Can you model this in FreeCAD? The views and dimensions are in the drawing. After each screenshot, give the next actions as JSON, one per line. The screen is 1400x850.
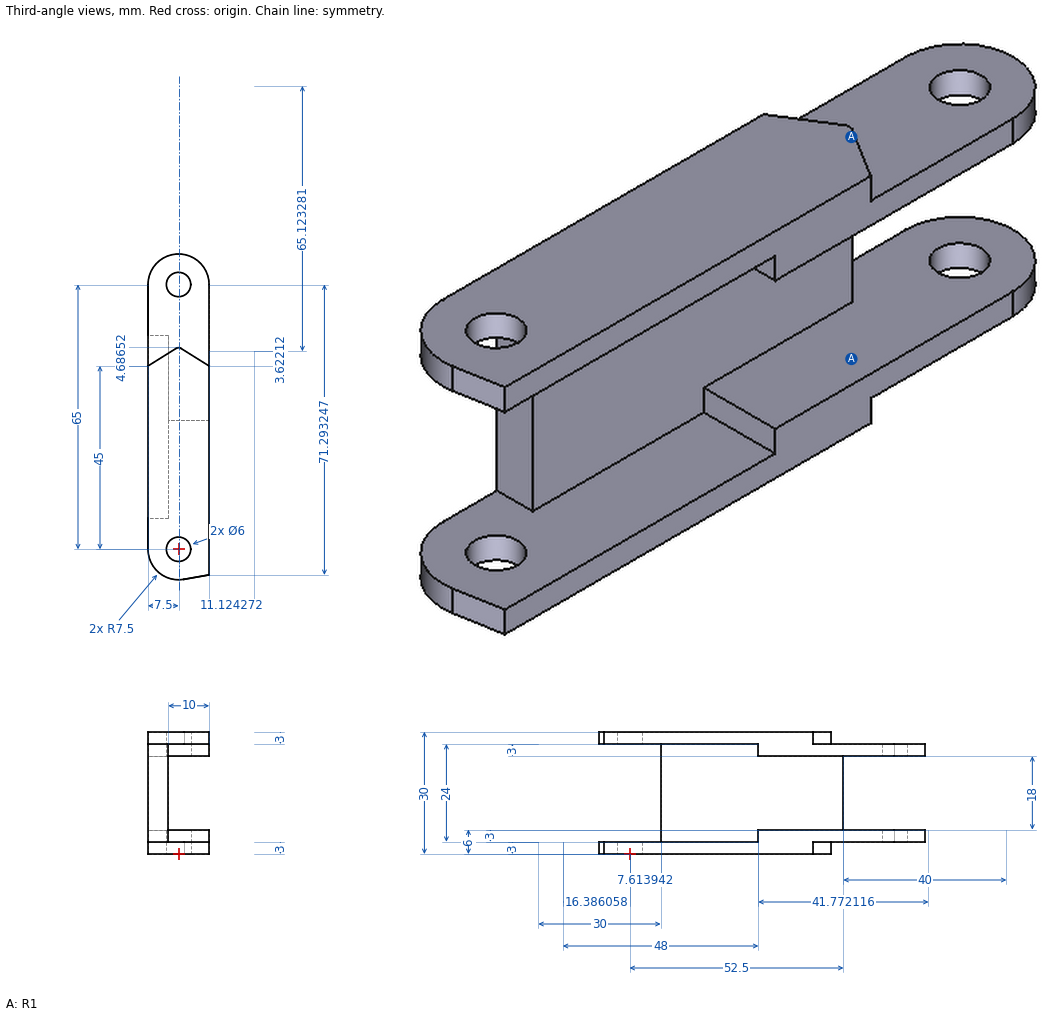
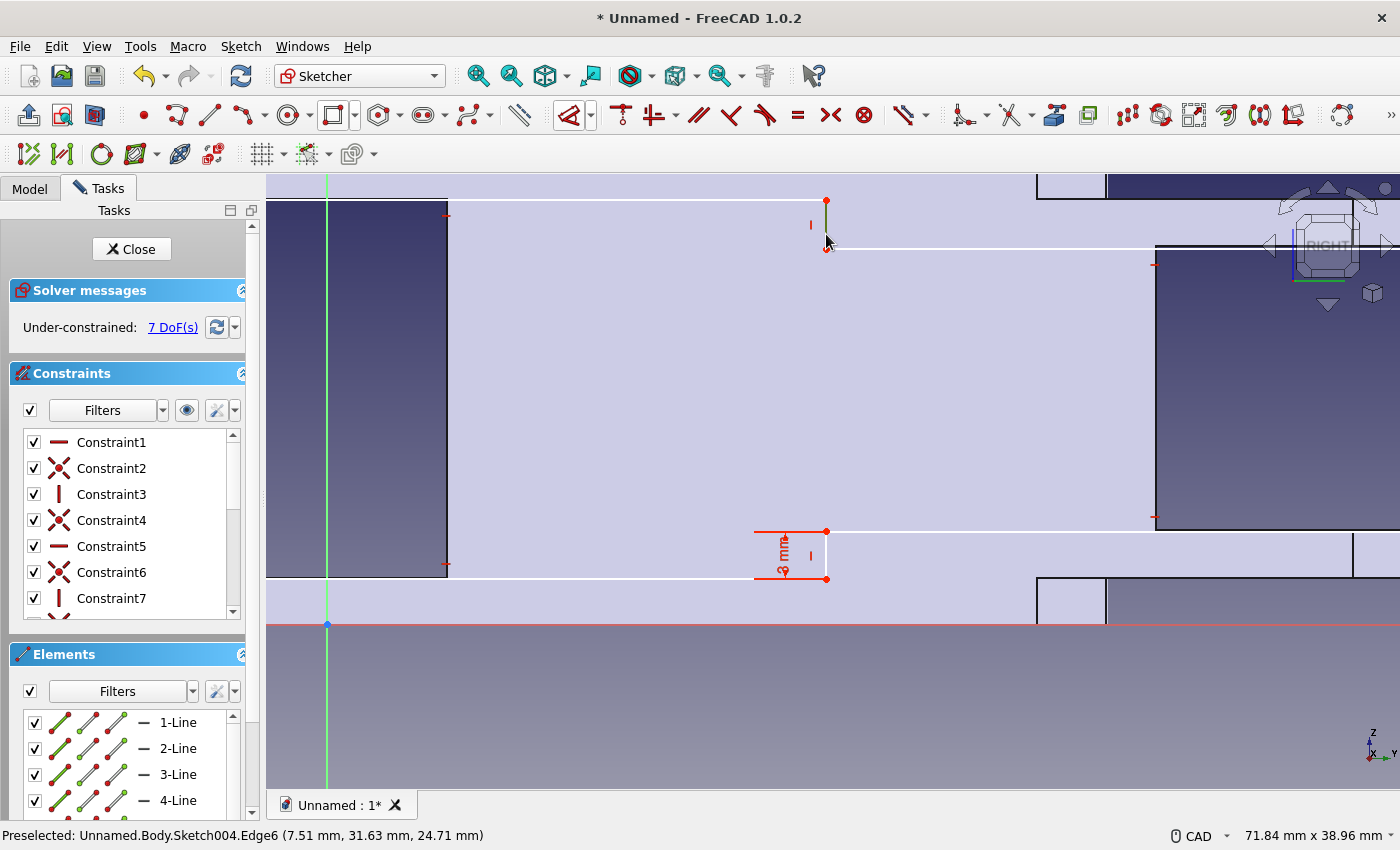
{"action": "key", "text": "i"}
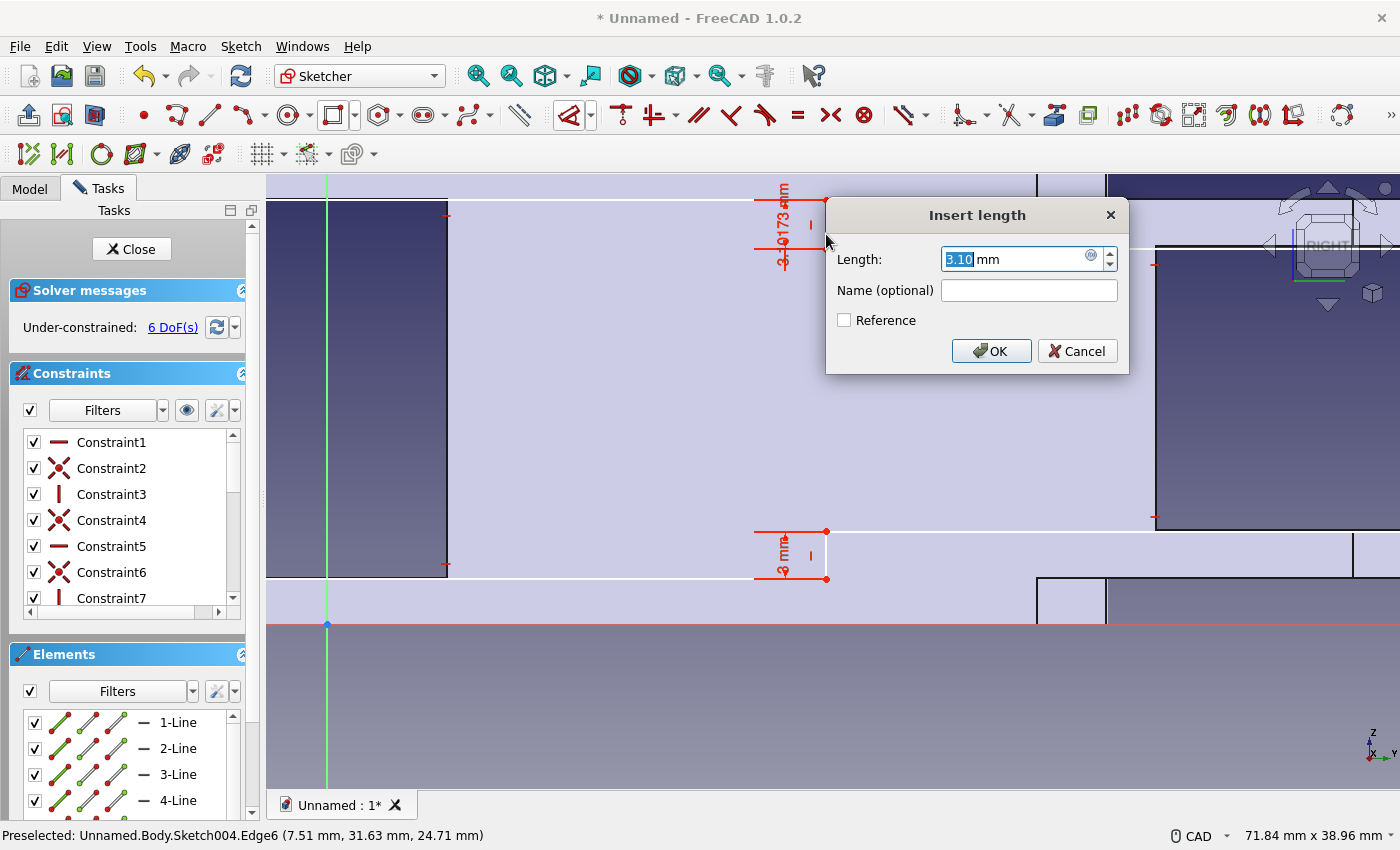
{"action": "type", "text": "3"}
{"action": "key", "text": "Return"}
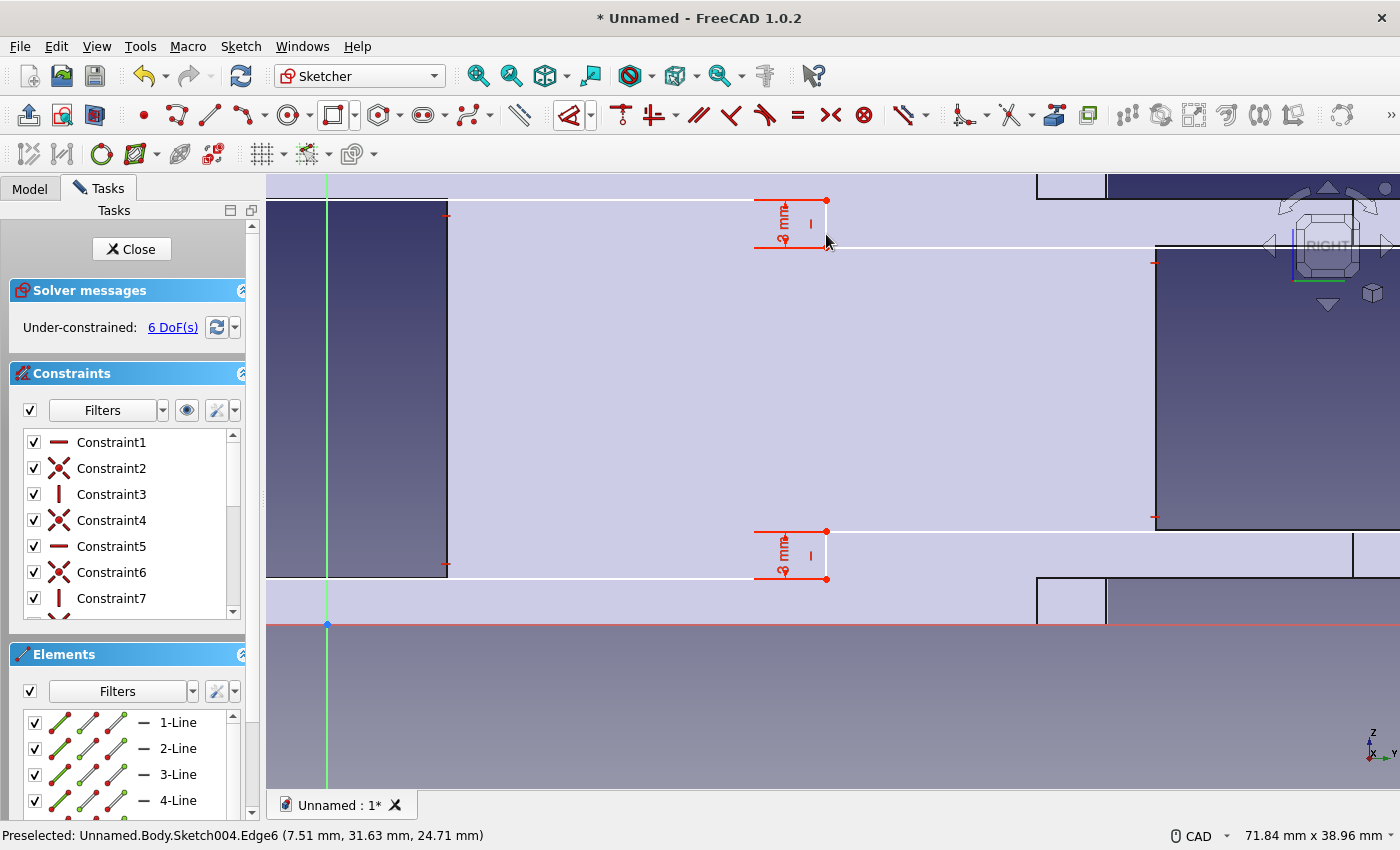
{"action": "left_click", "coordinate": [295, 579]}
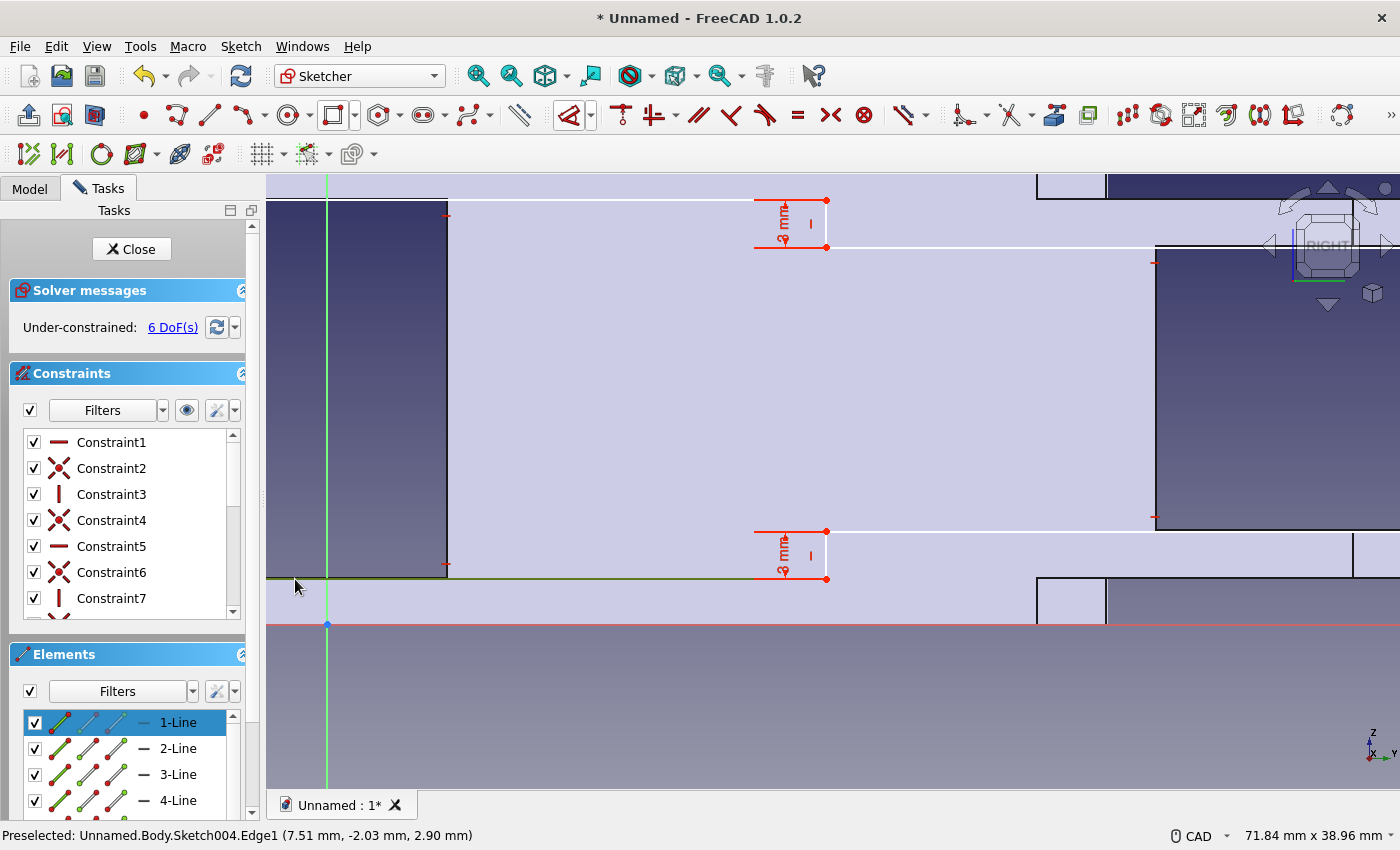
{"action": "key", "text": "l"}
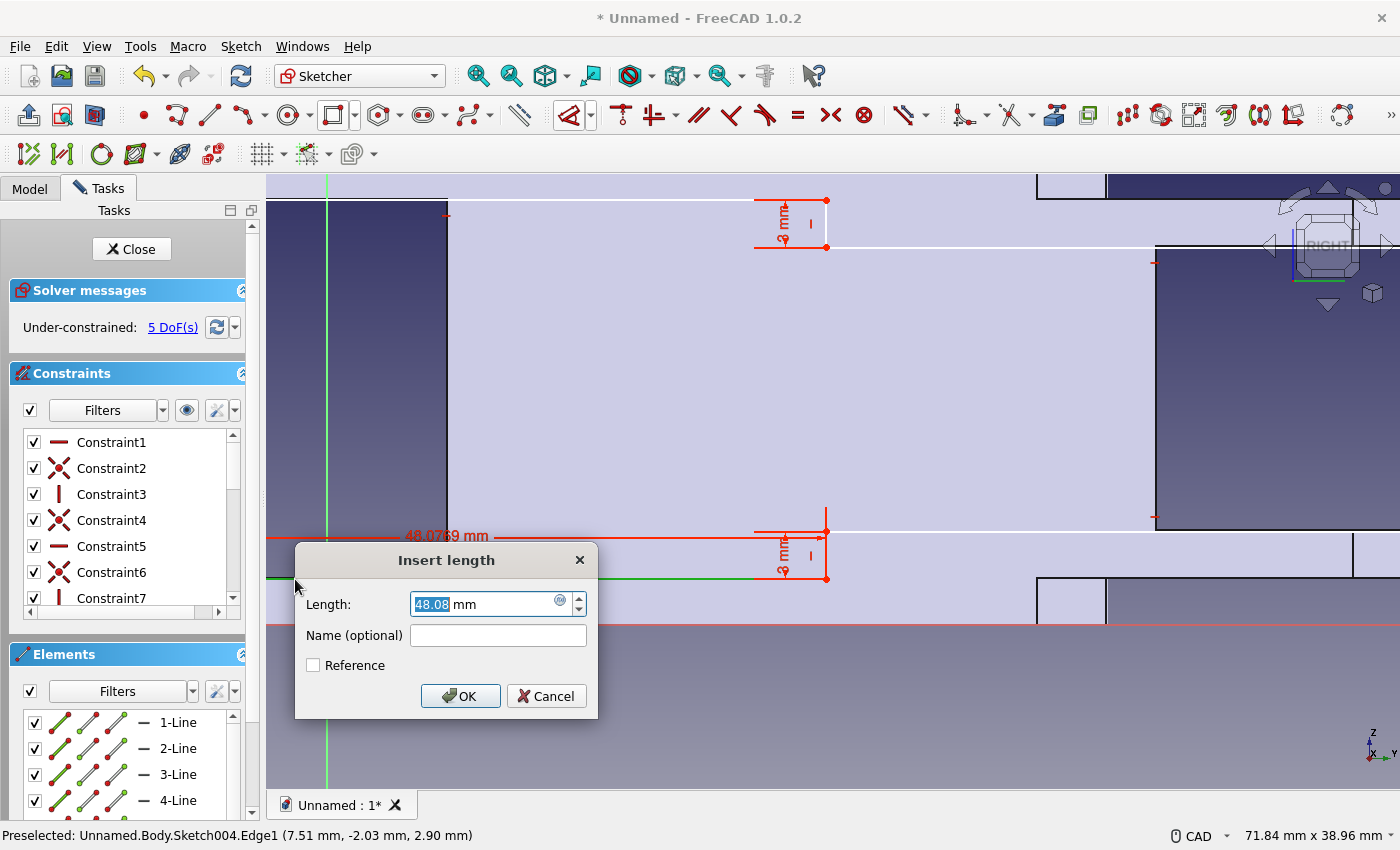
{"action": "type", "text": "48"}
{"action": "key", "text": "Return"}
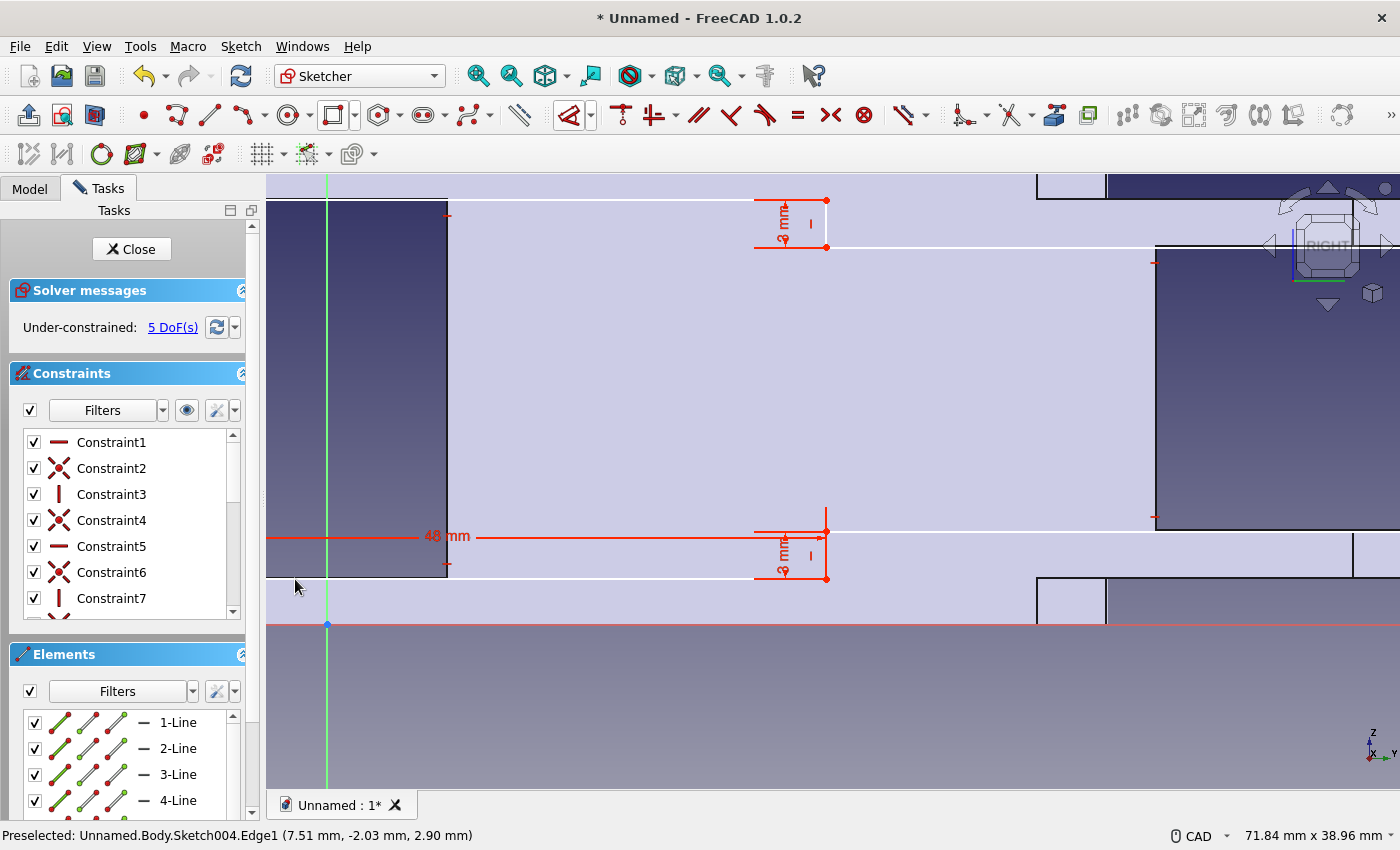
{"action": "scroll", "coordinate": [754, 538], "scroll_direction": "down", "scroll_amount": 4}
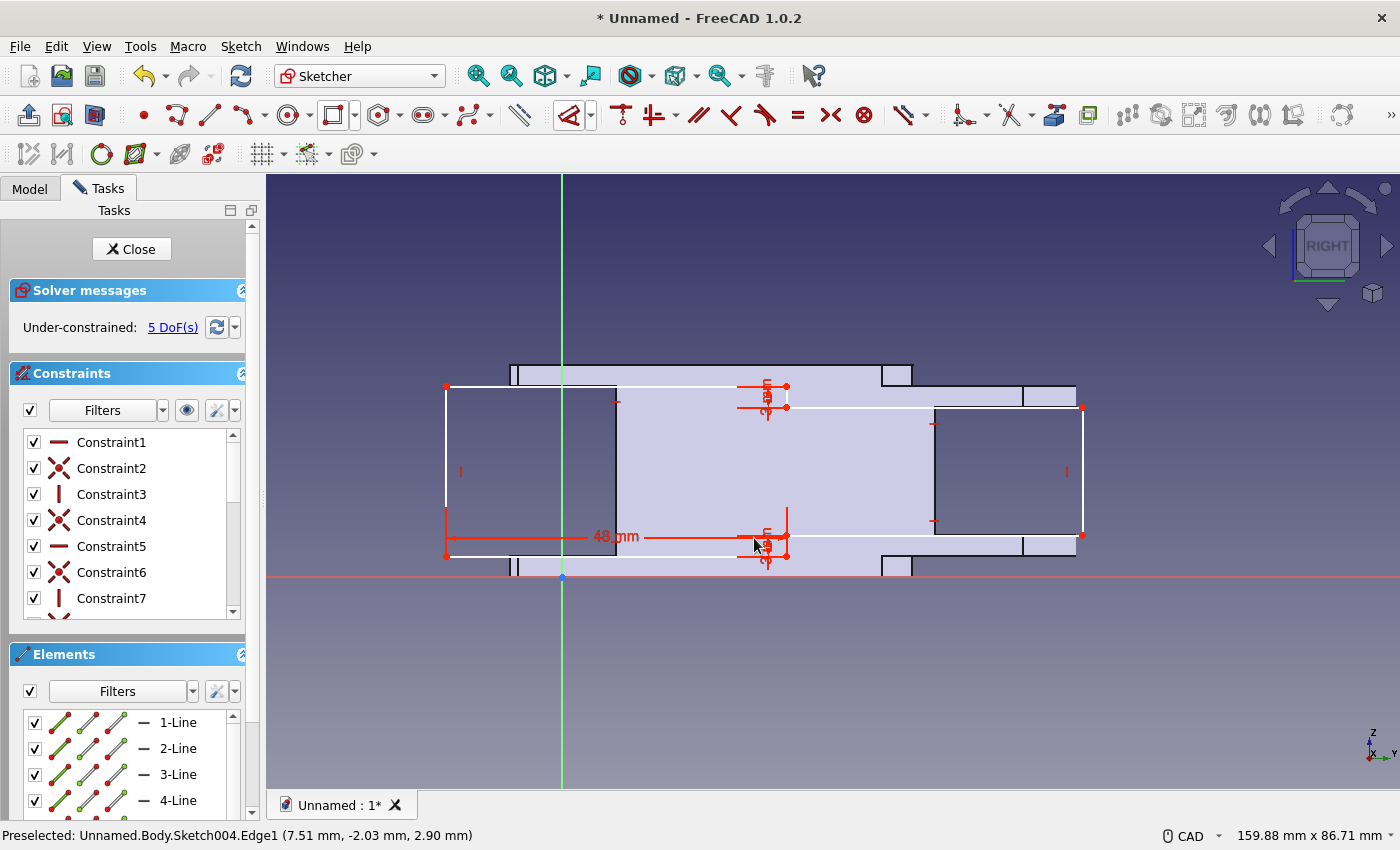
{"action": "left_click", "coordinate": [1083, 497]}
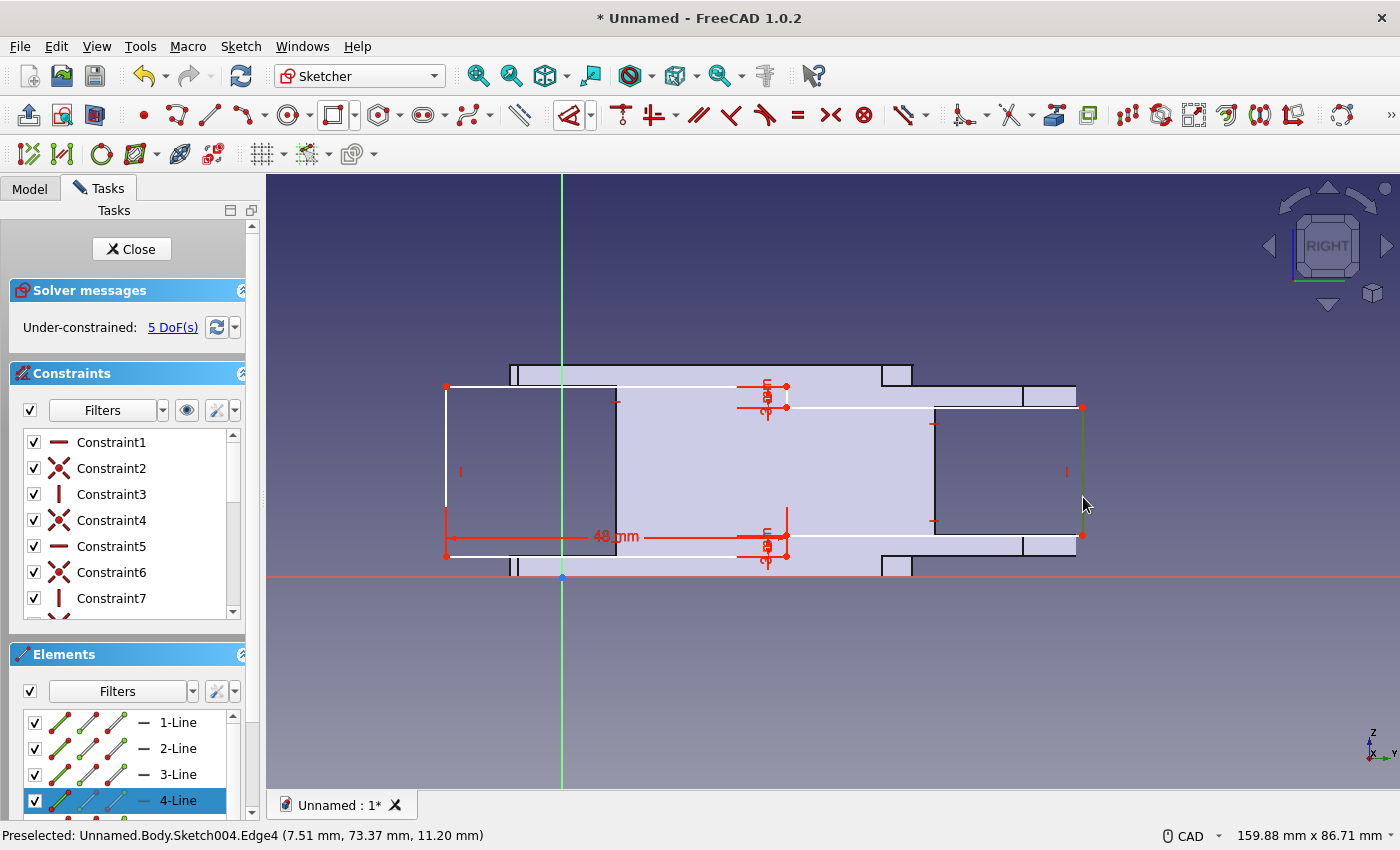
{"action": "key", "text": "i"}